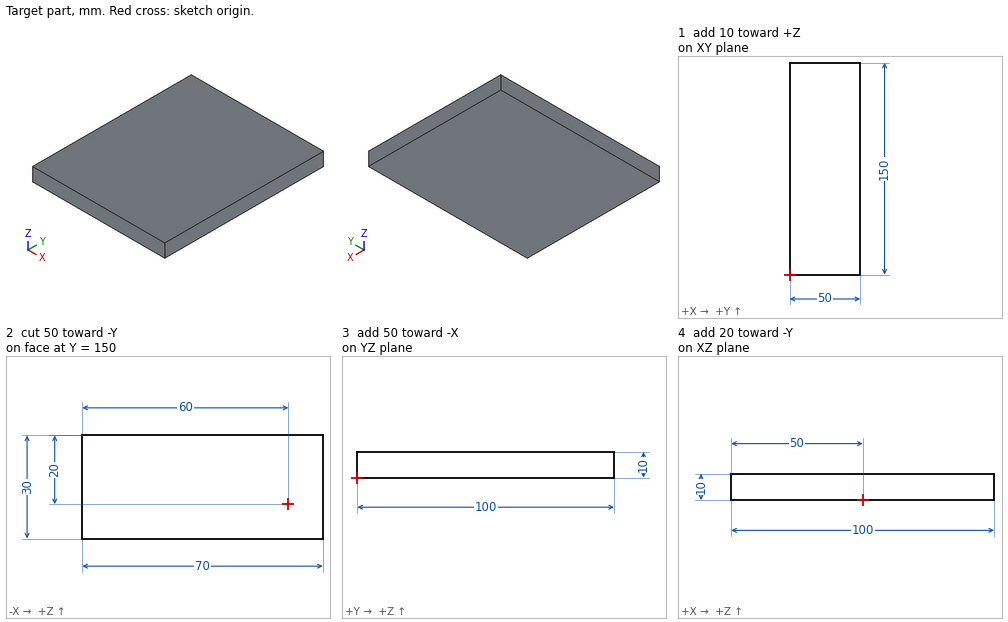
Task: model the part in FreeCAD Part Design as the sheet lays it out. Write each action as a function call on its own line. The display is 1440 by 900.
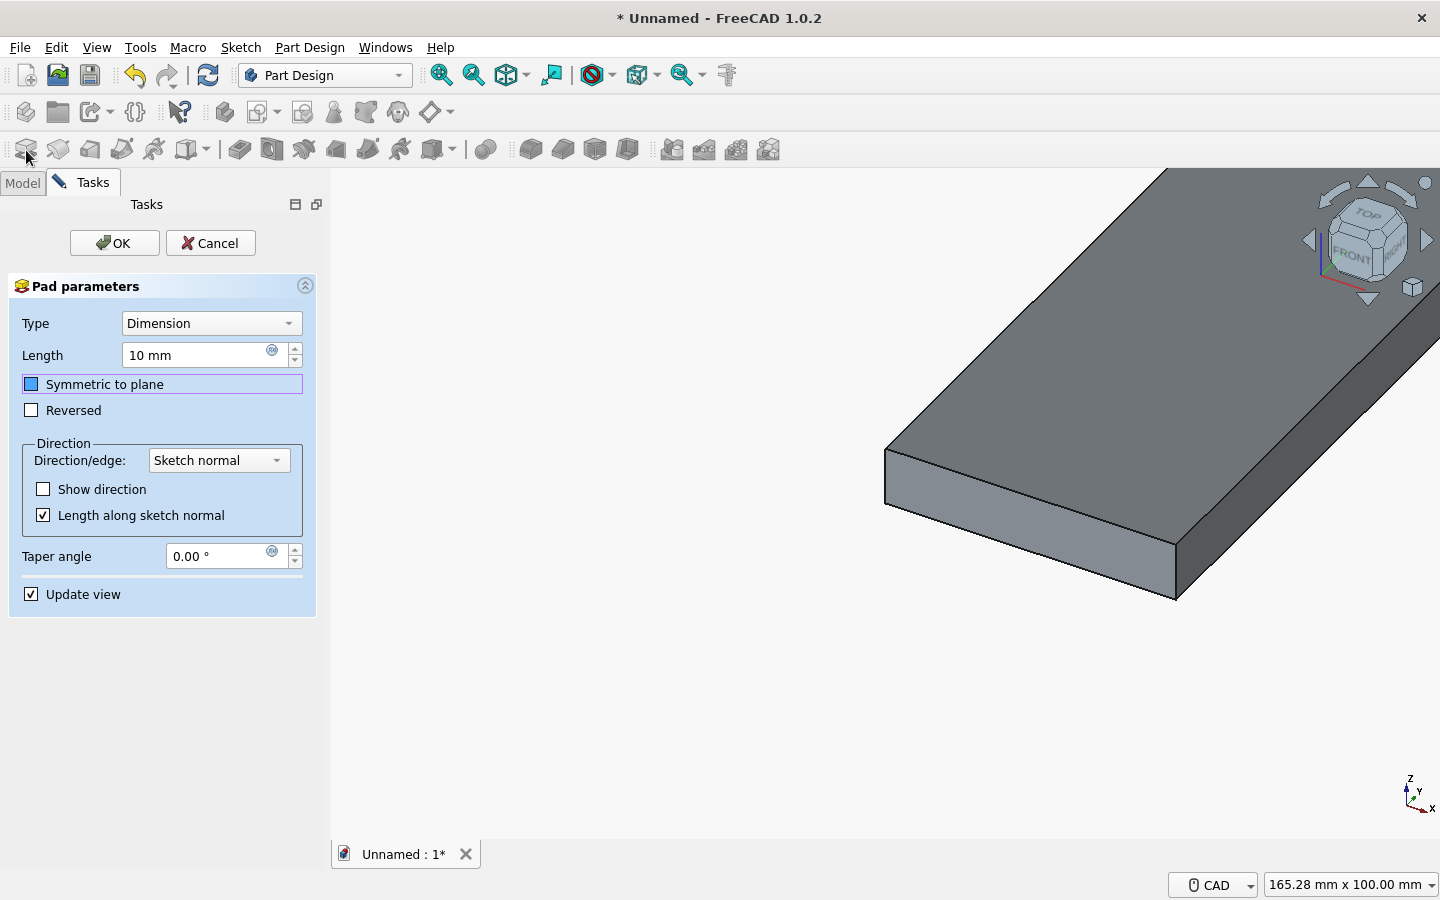
click(115, 243)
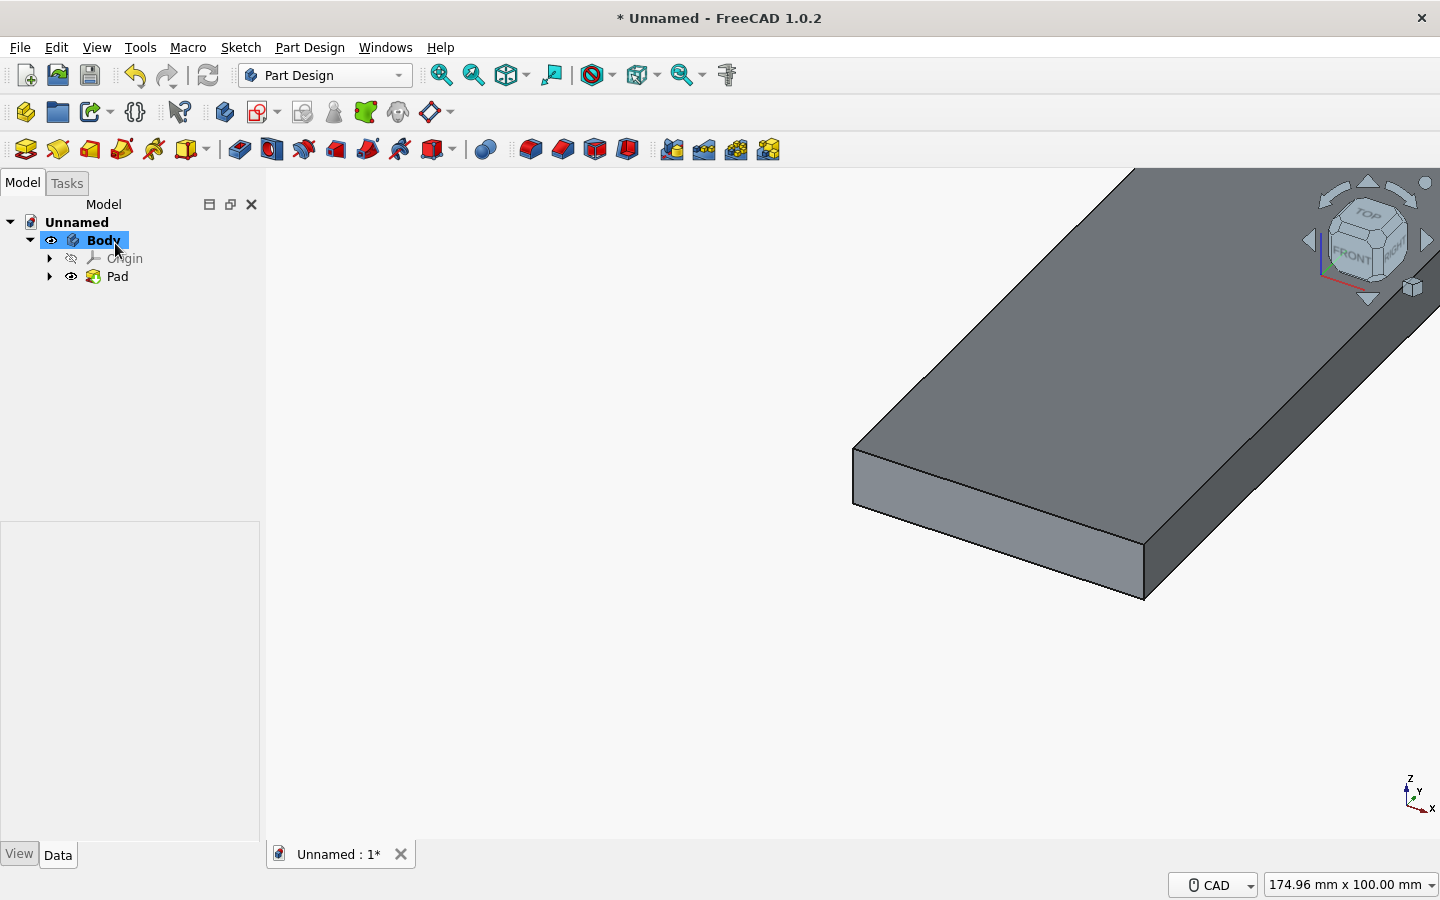
click(442, 76)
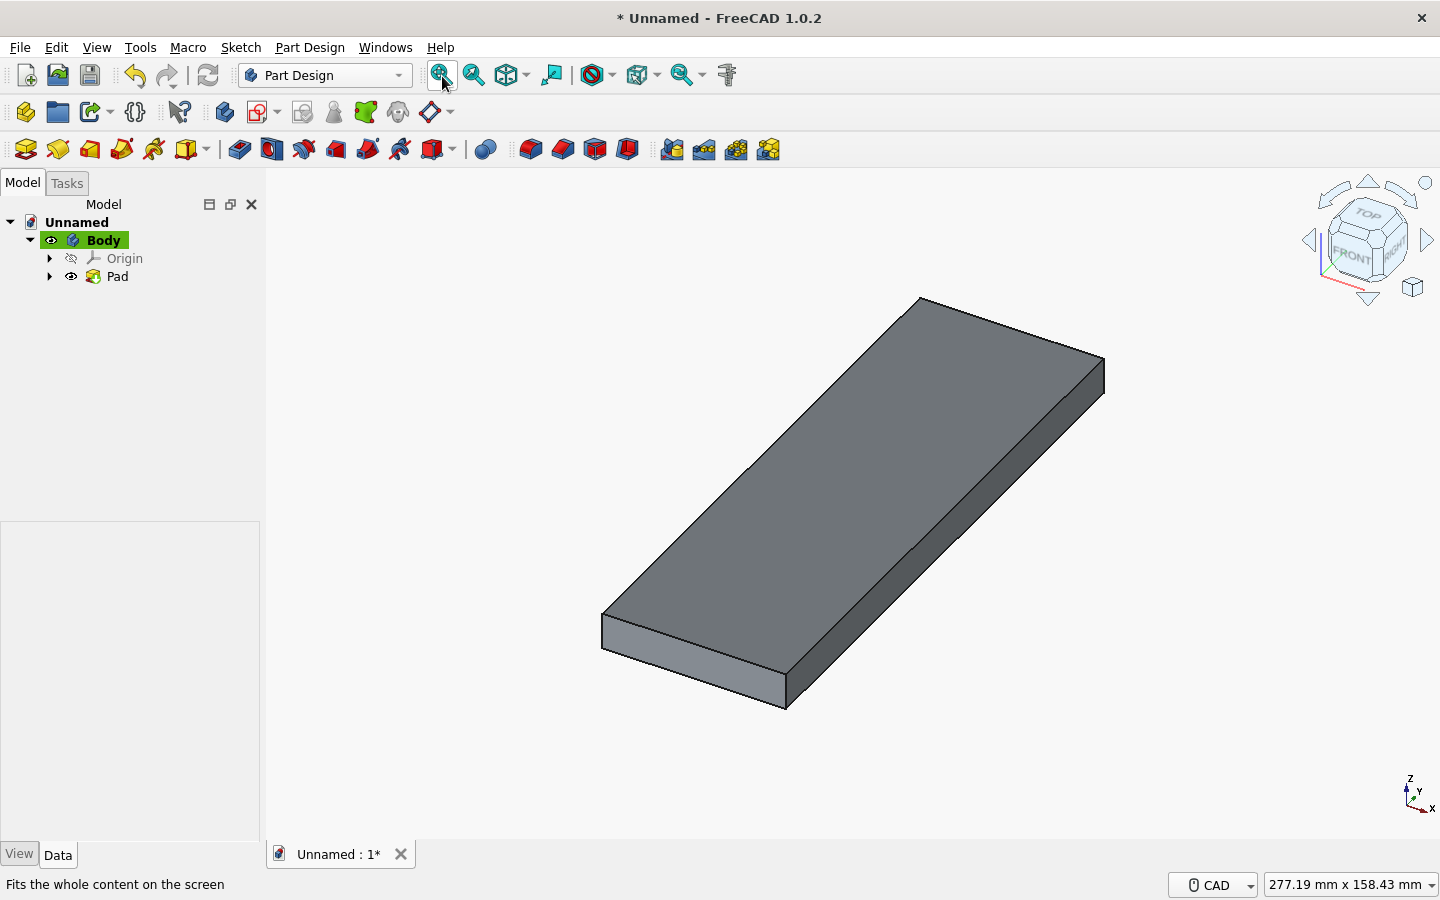
key(4)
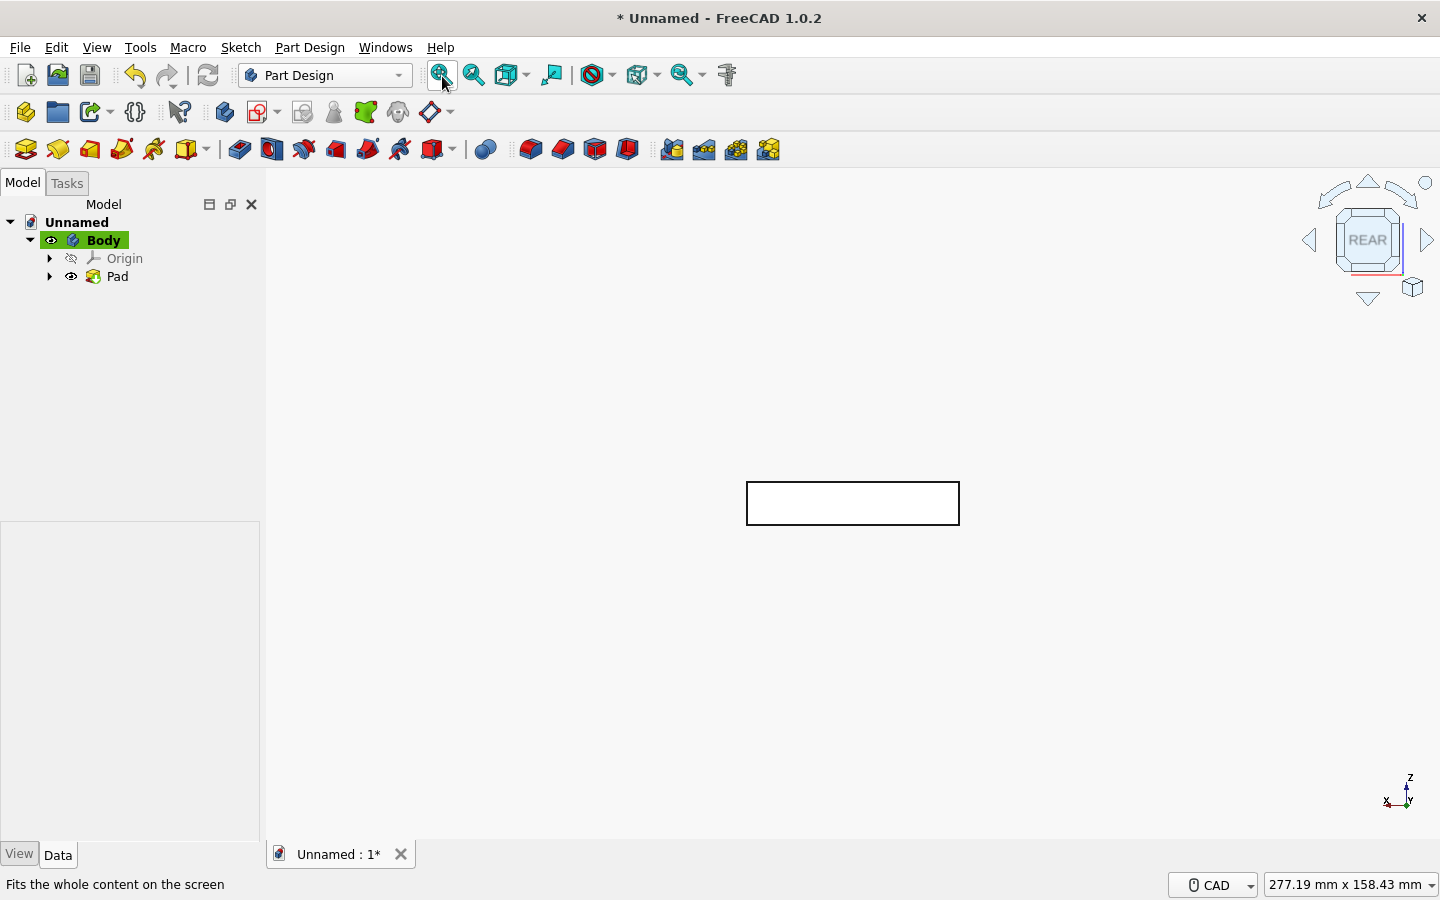
click(442, 76)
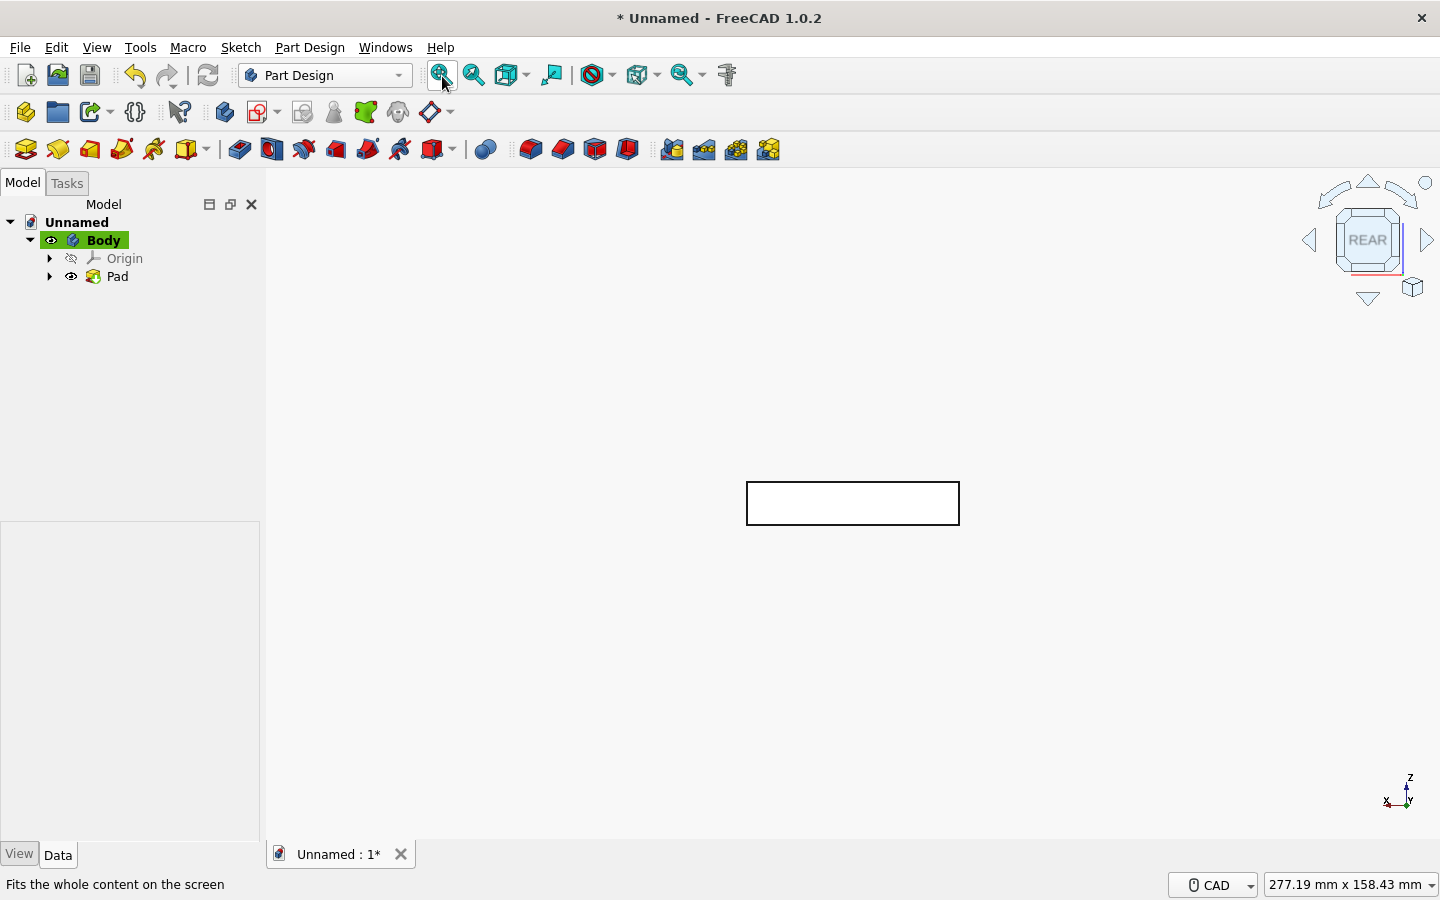
click(792, 503)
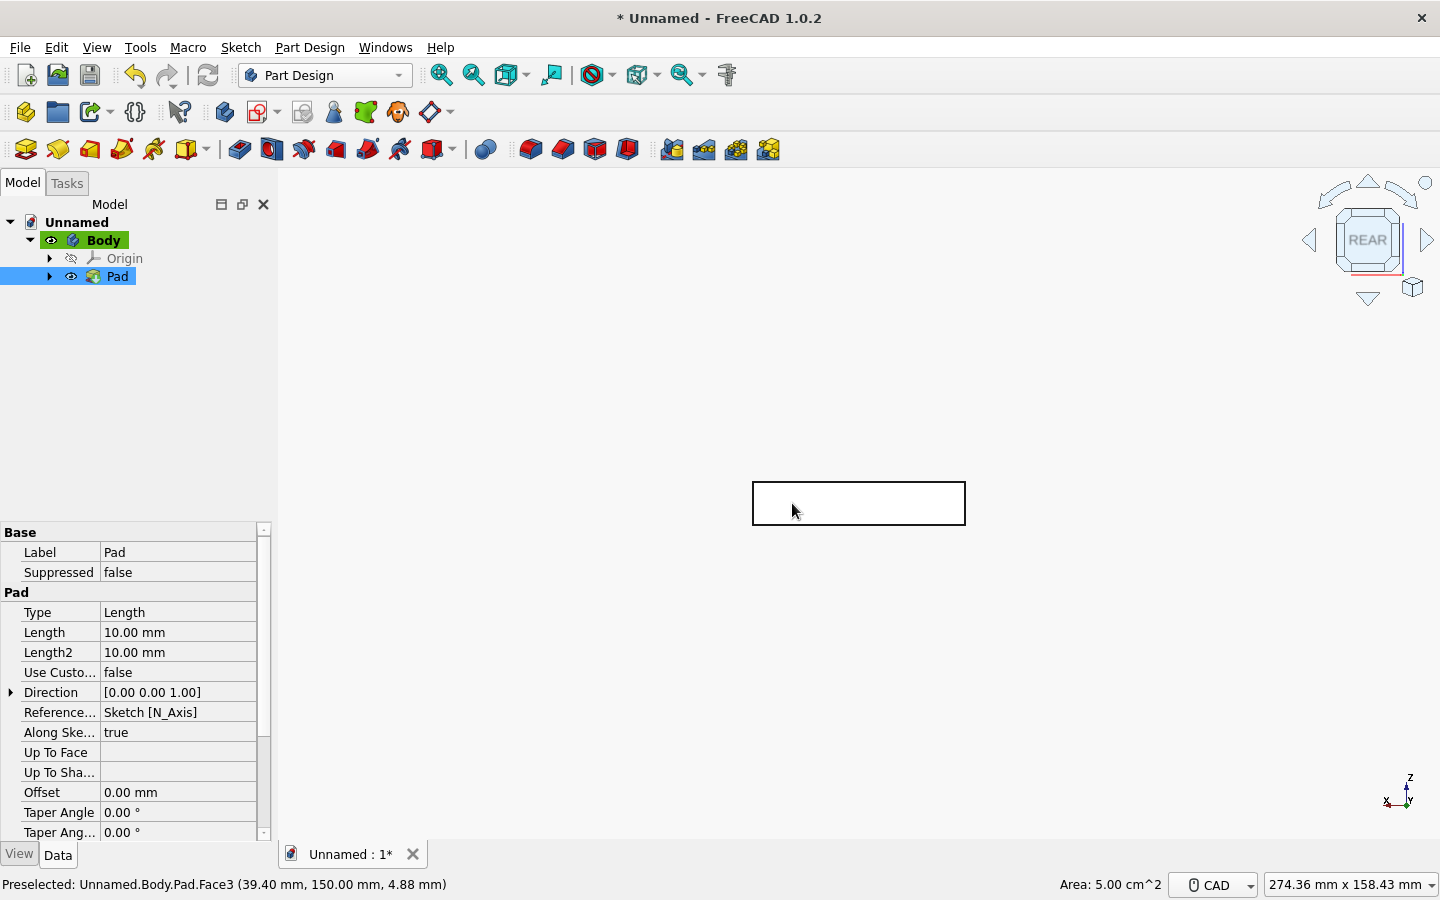
click(258, 112)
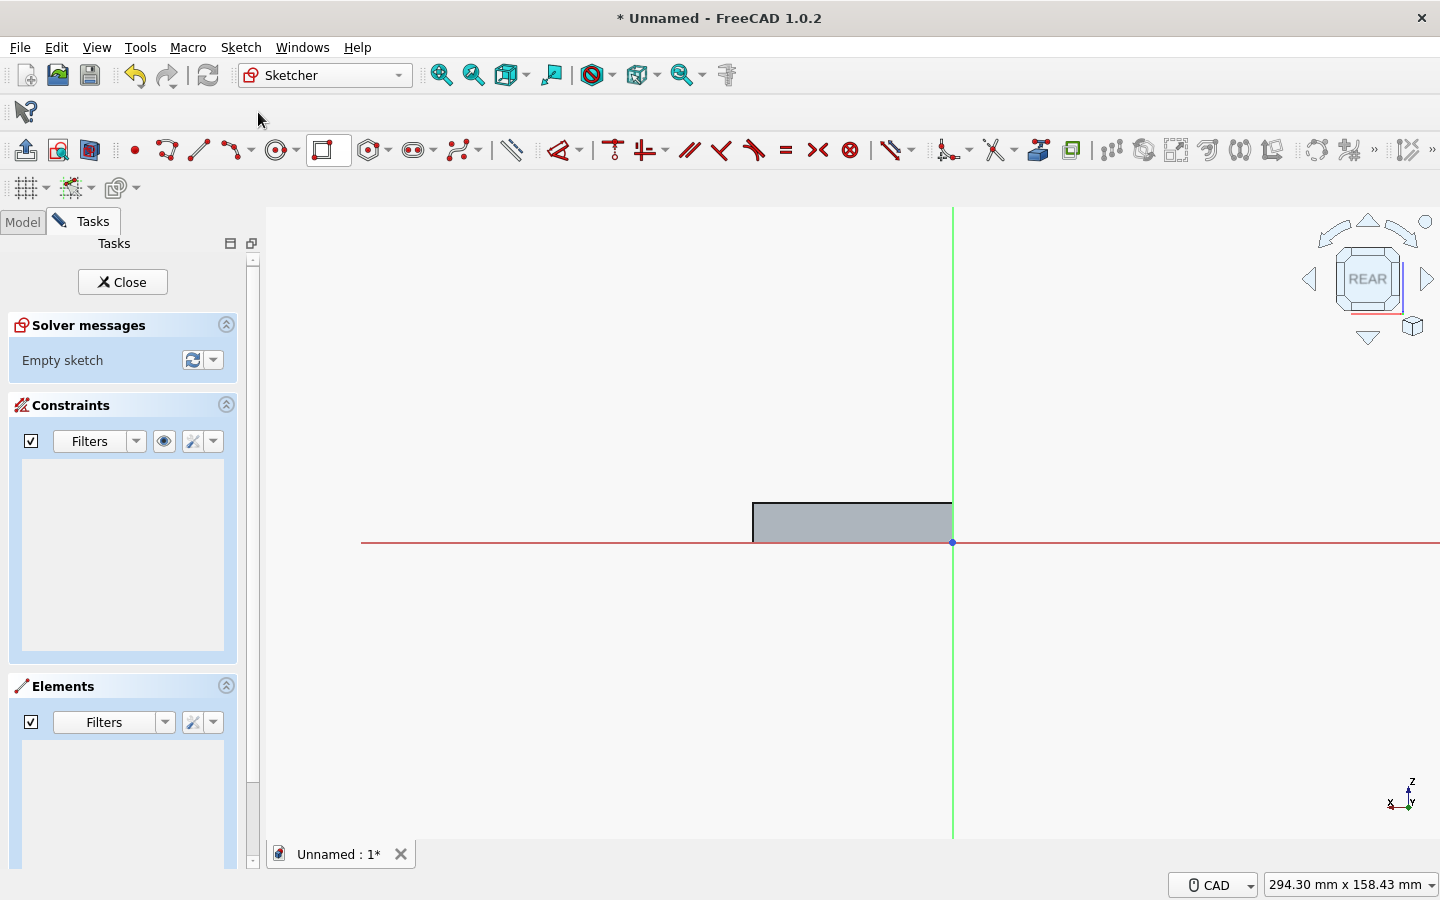
scroll(893, 523, up, 5)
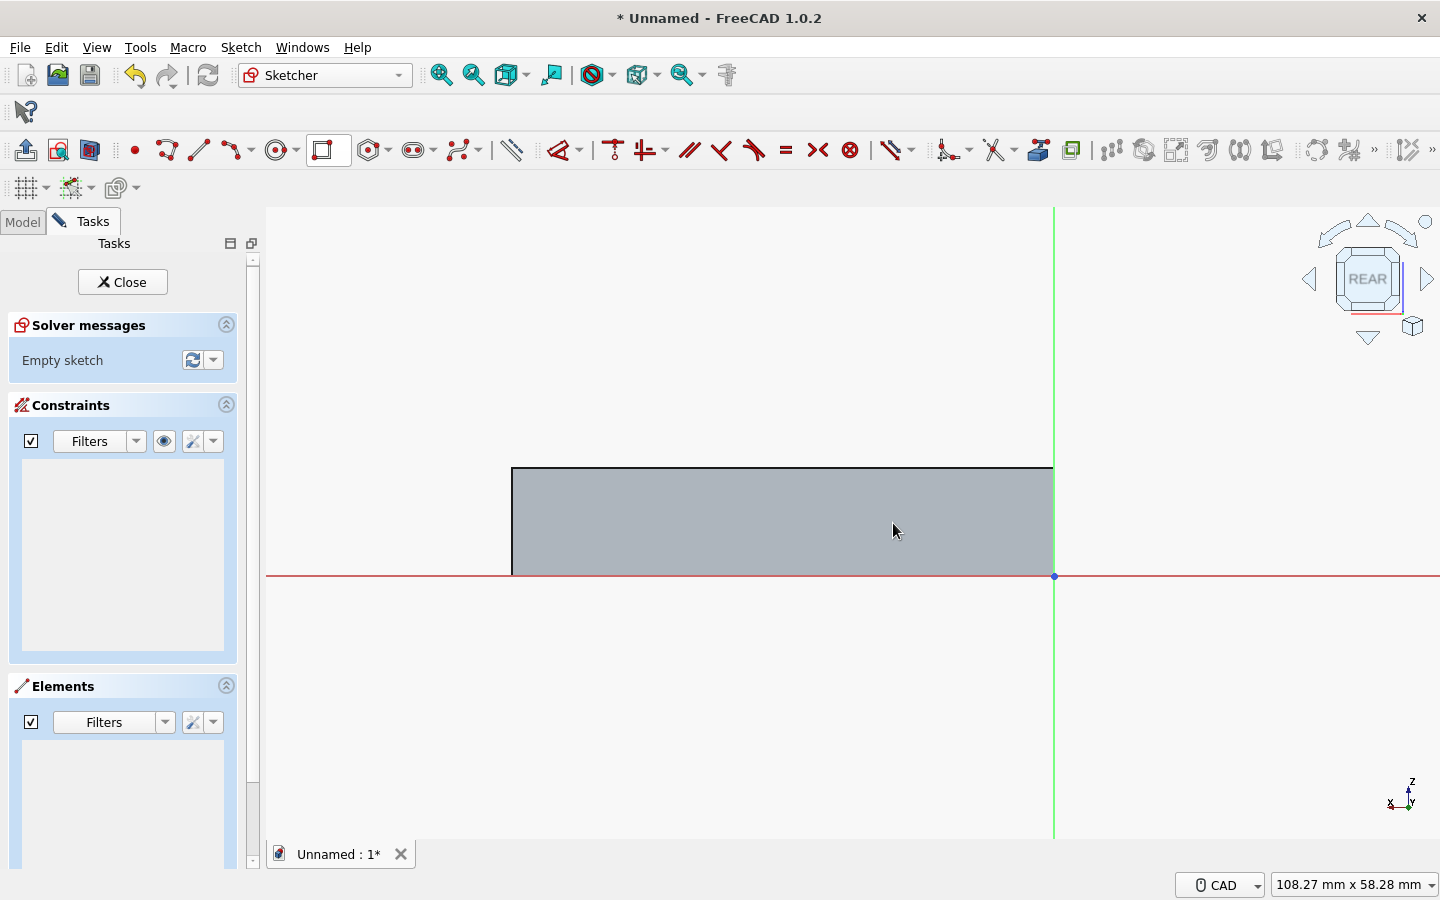
click(322, 150)